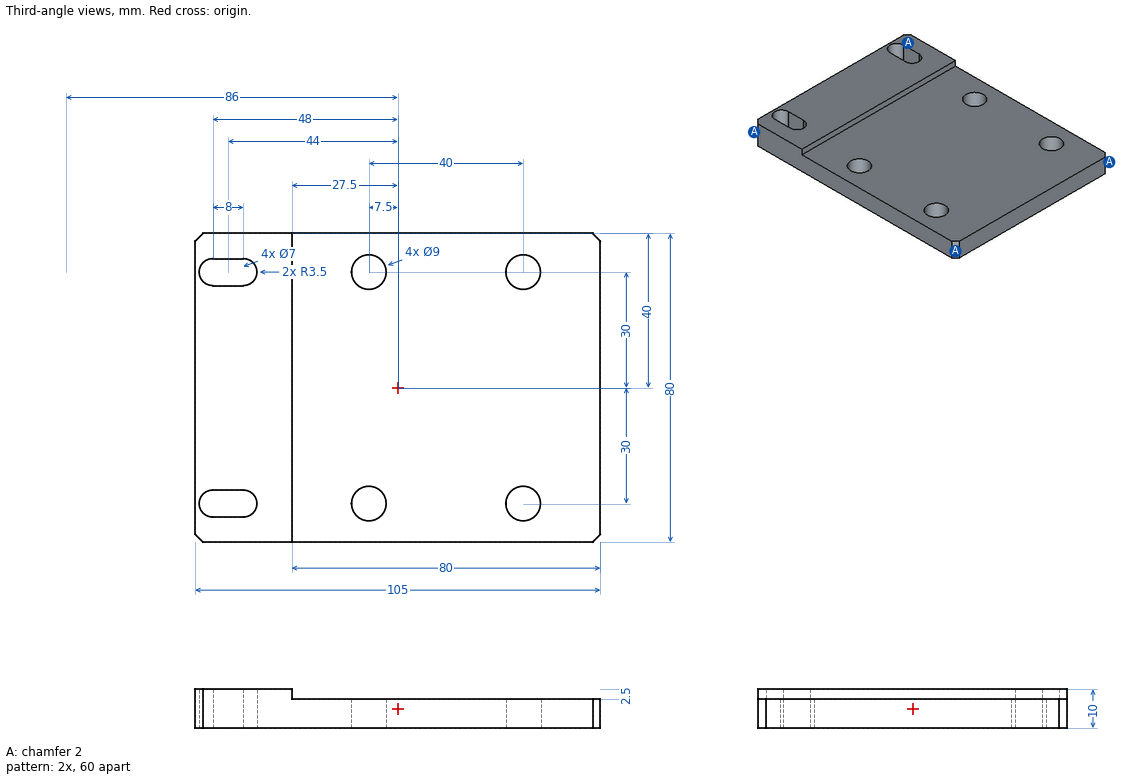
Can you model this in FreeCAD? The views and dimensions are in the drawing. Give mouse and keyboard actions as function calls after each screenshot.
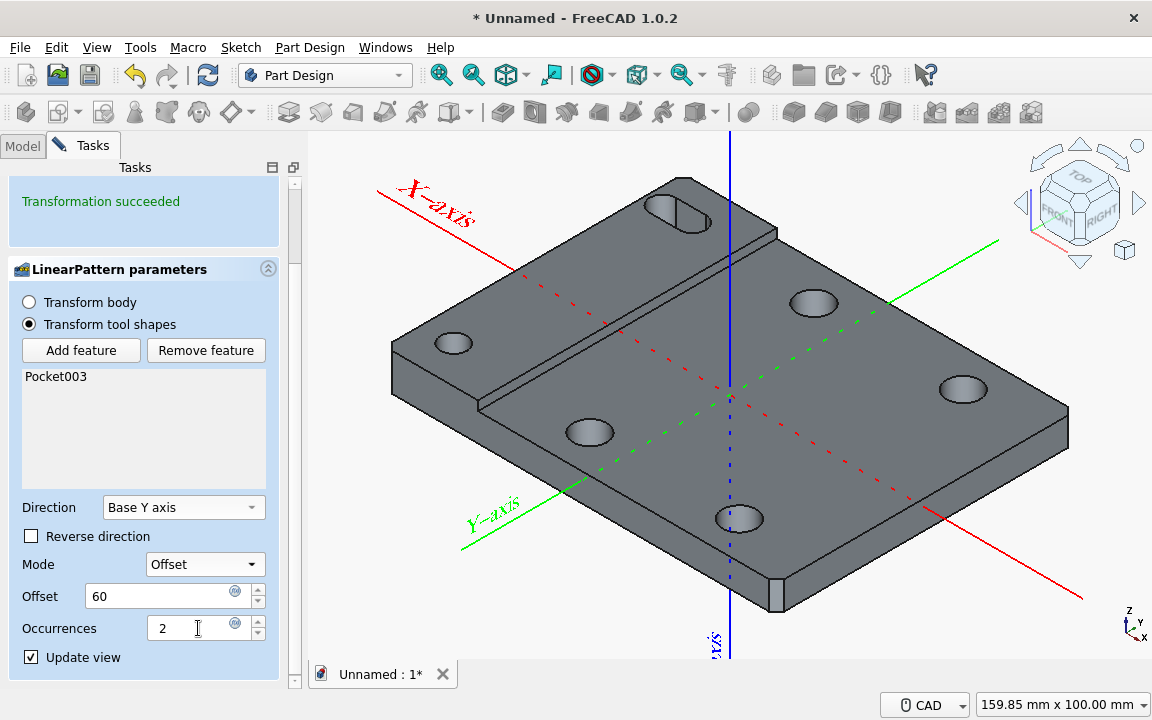
click(30, 536)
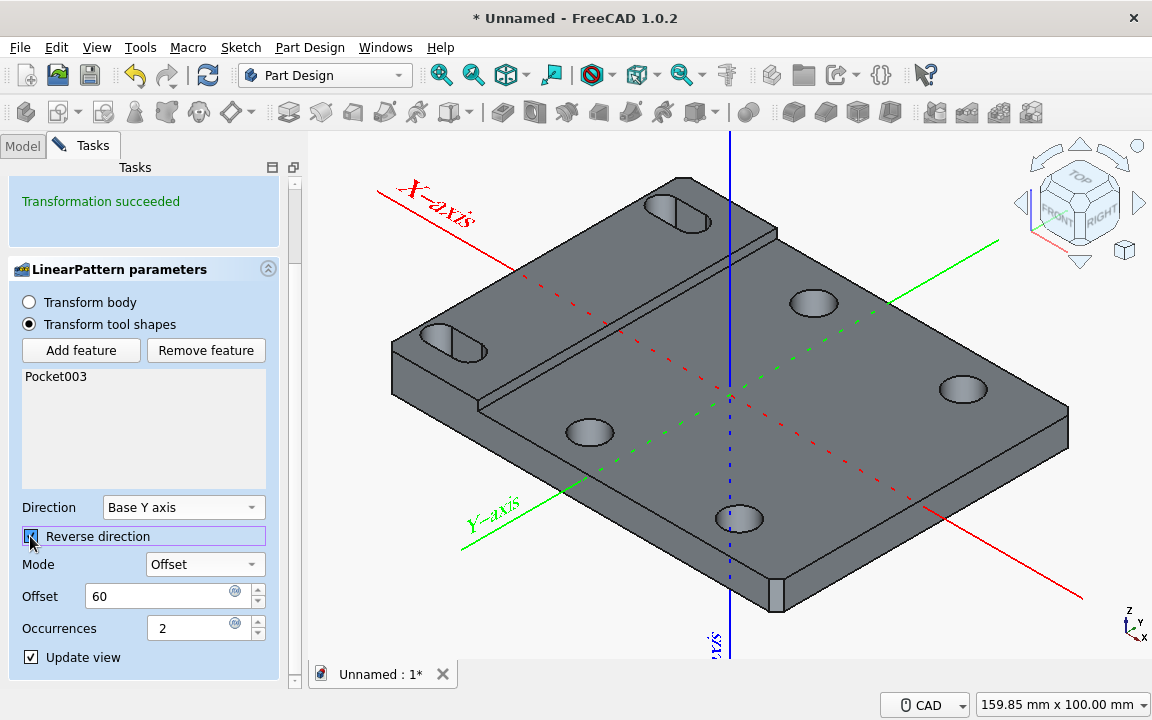
scroll(295, 432, up, 3)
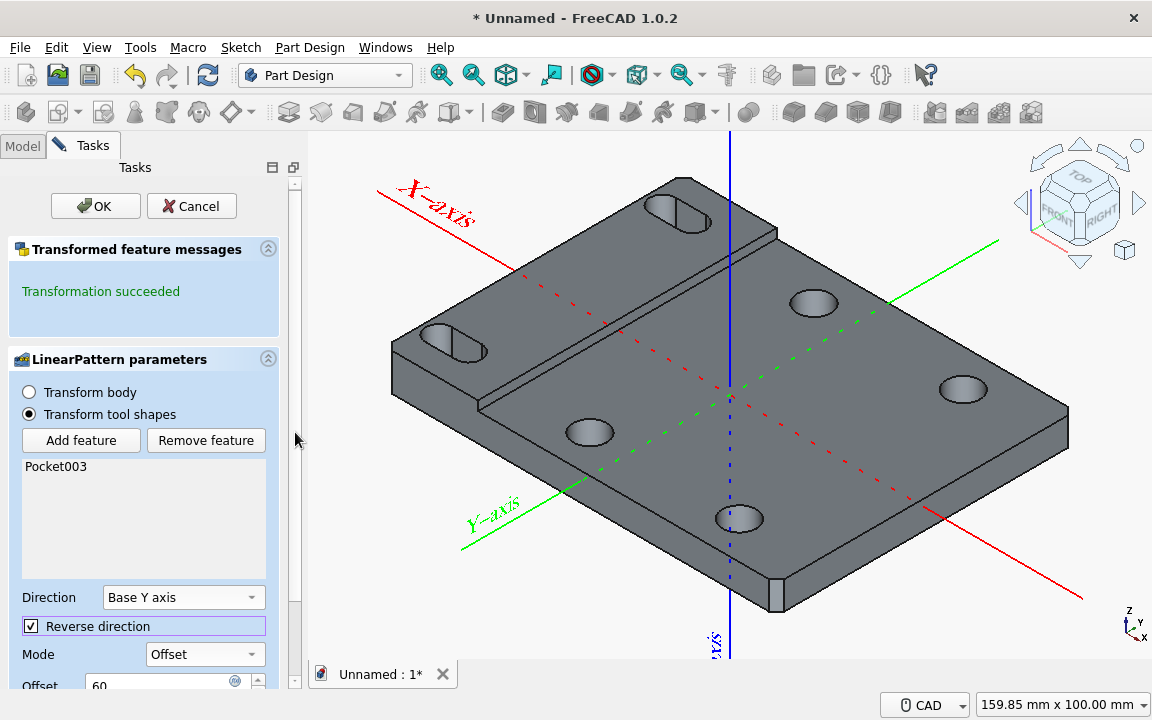
click(96, 206)